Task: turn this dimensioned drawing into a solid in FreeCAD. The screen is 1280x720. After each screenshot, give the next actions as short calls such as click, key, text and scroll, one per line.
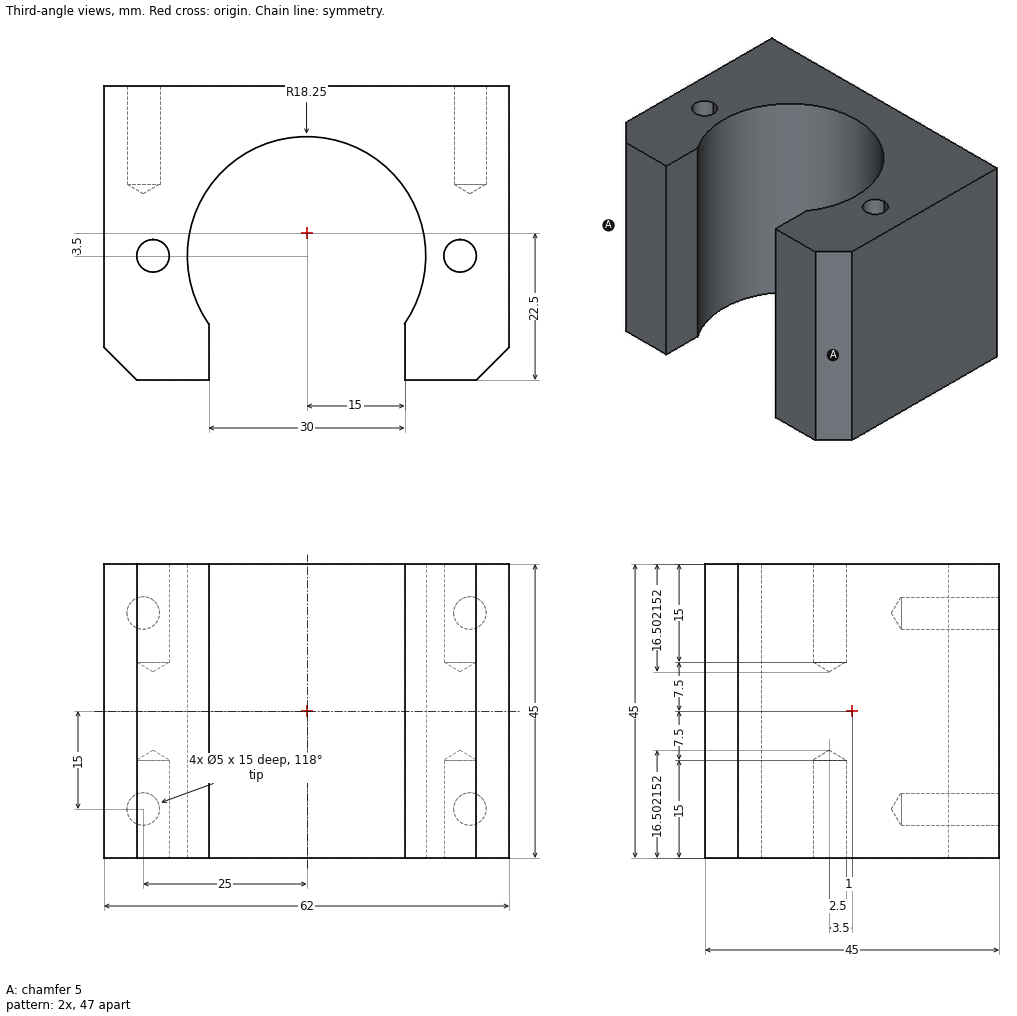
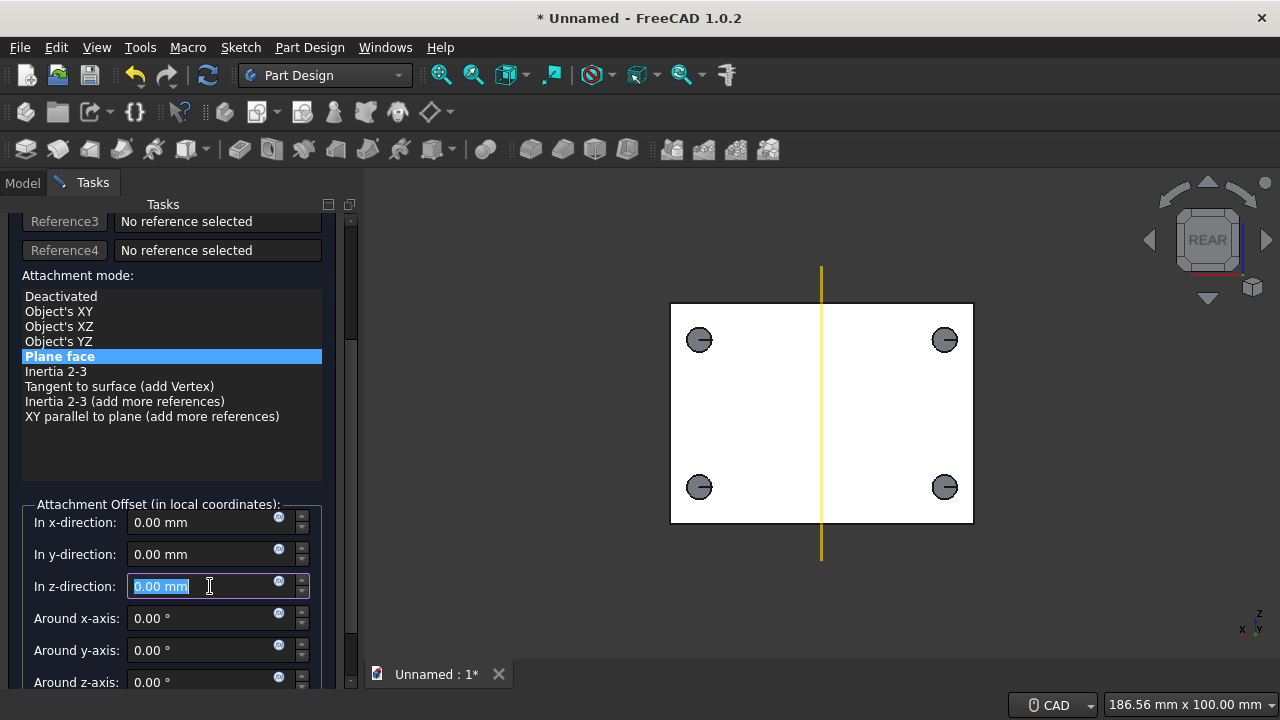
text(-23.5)
key(Tab)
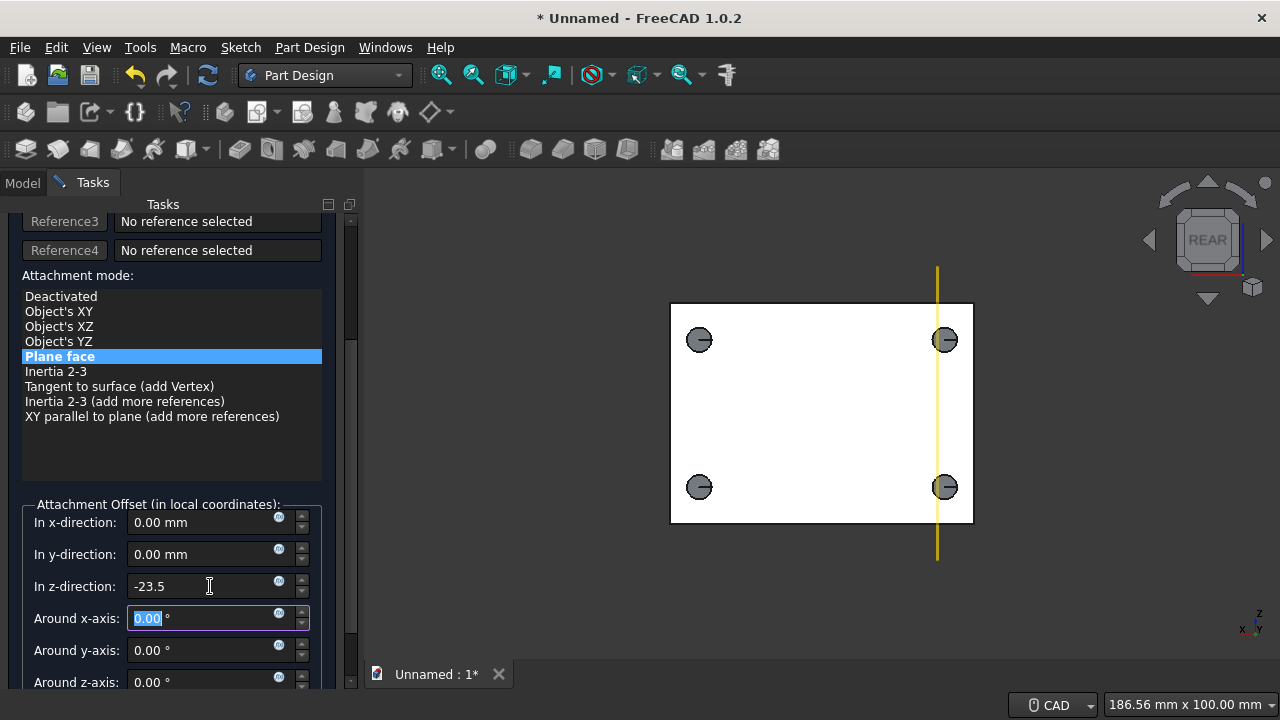
scroll(351, 451, up, 4)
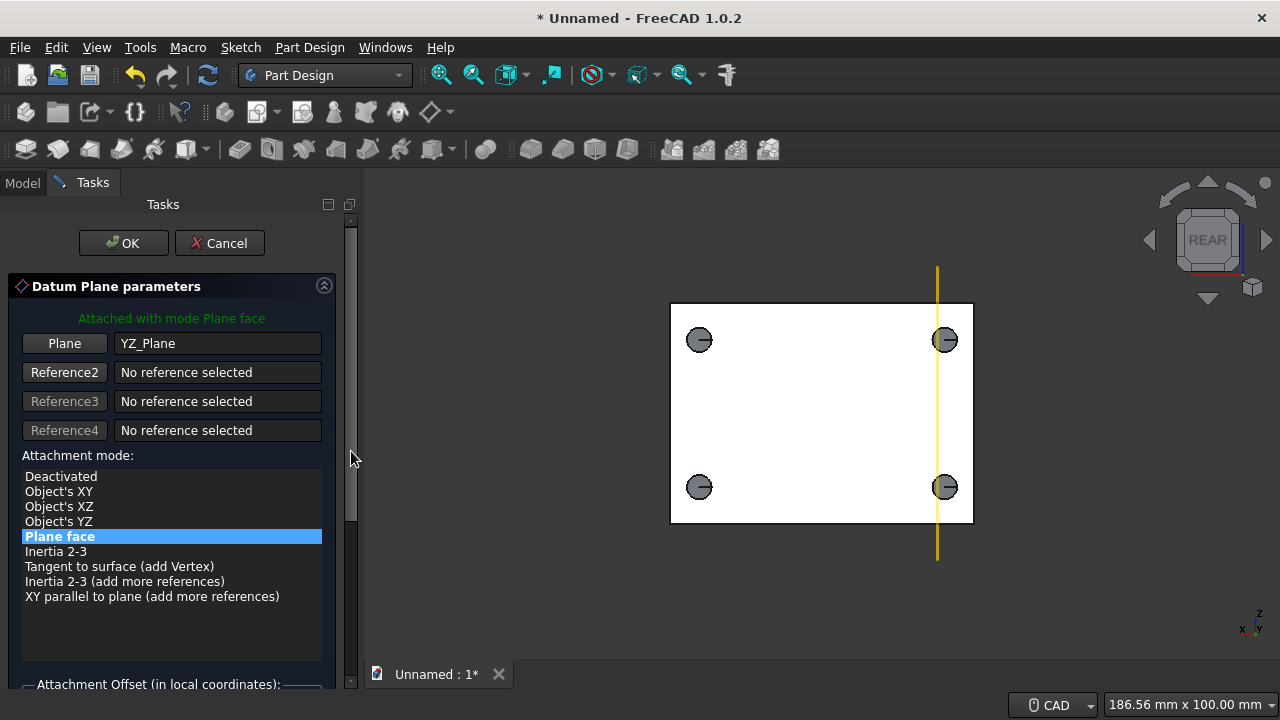
click(124, 243)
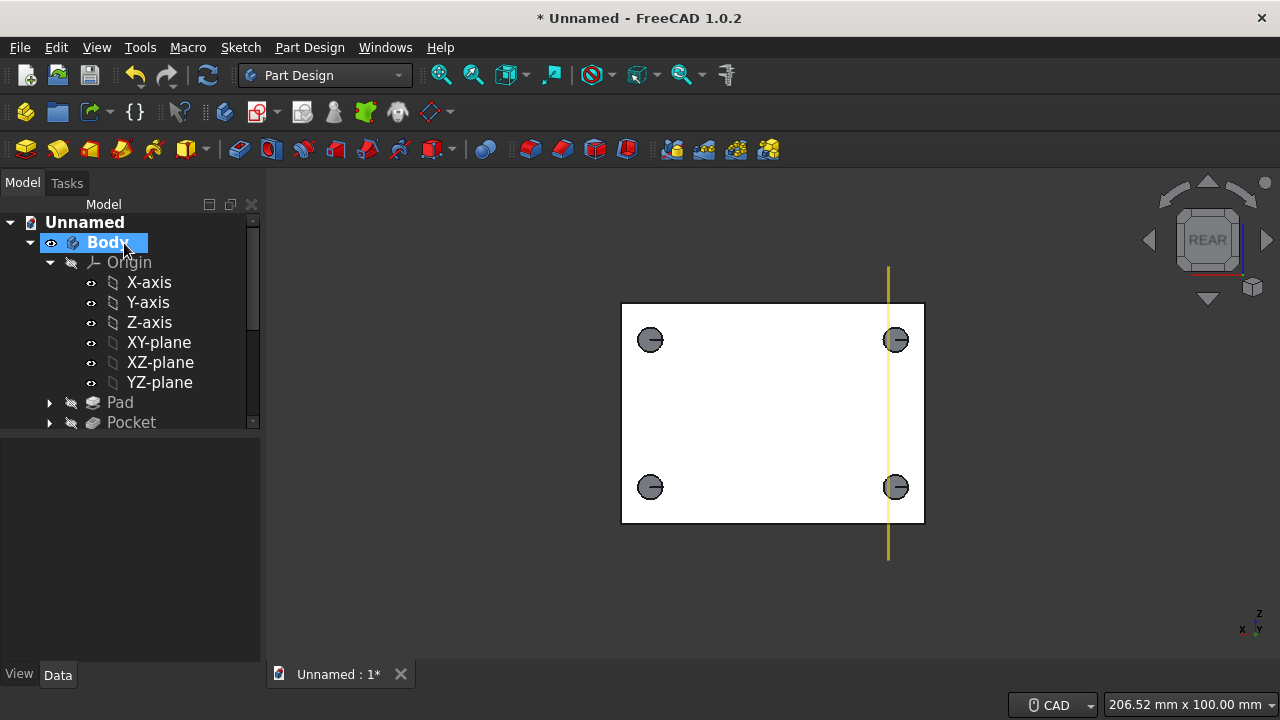
scroll(100, 318, down, 3)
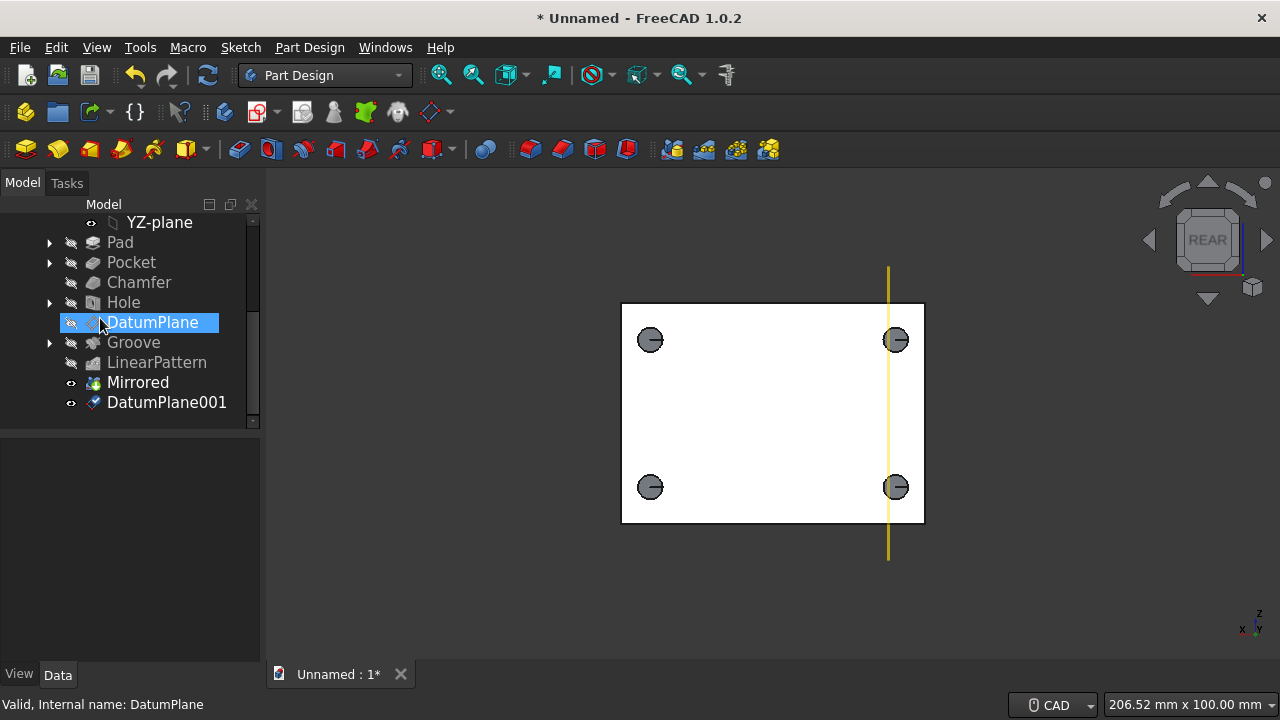
click(116, 403)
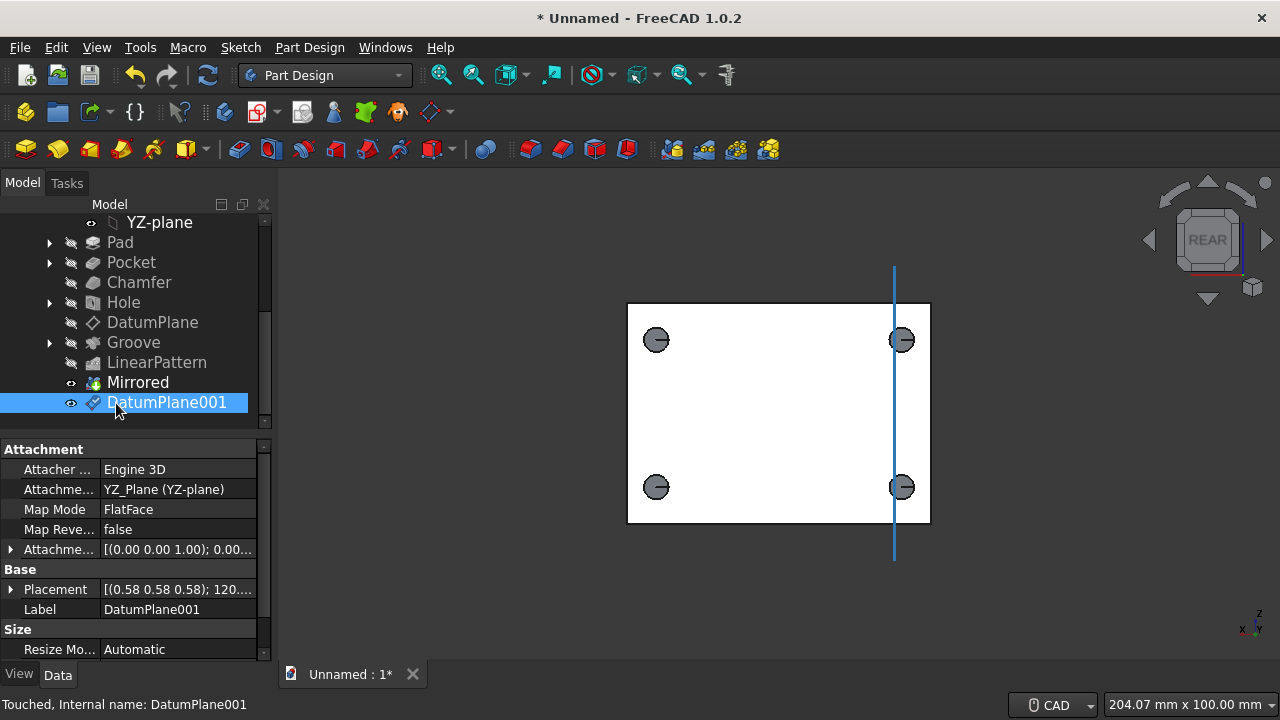
click(258, 112)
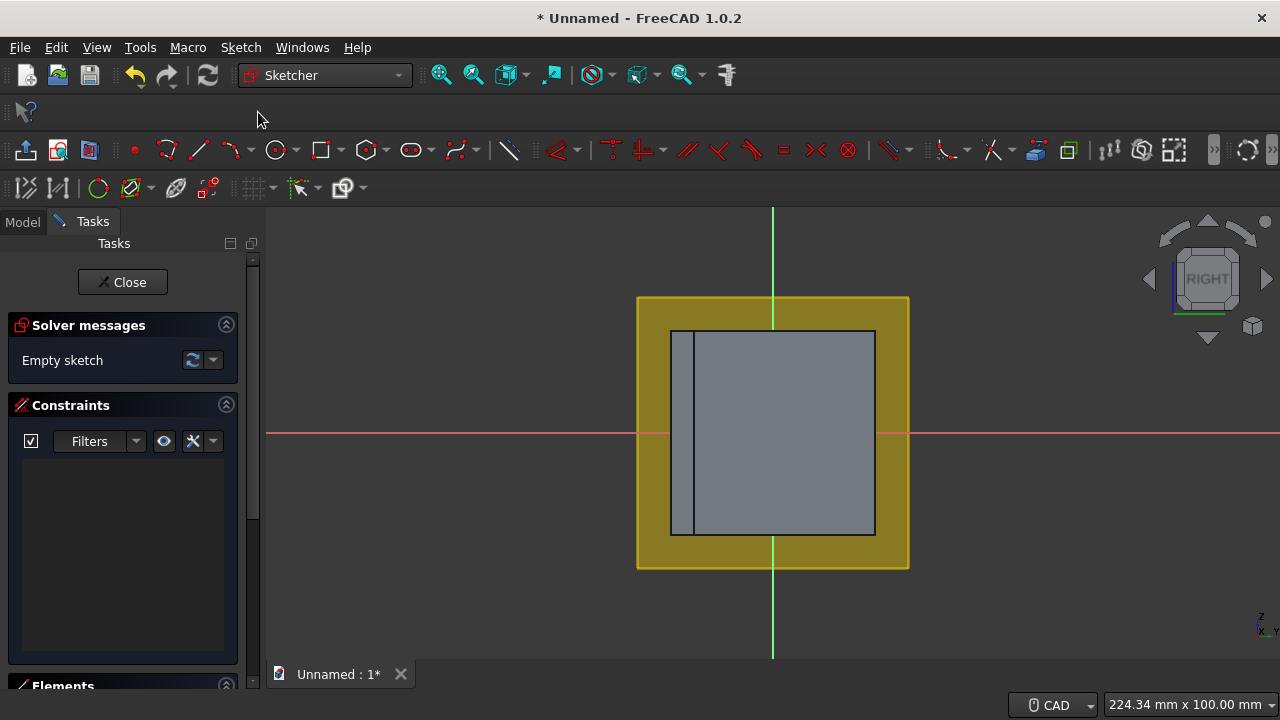
click(90, 150)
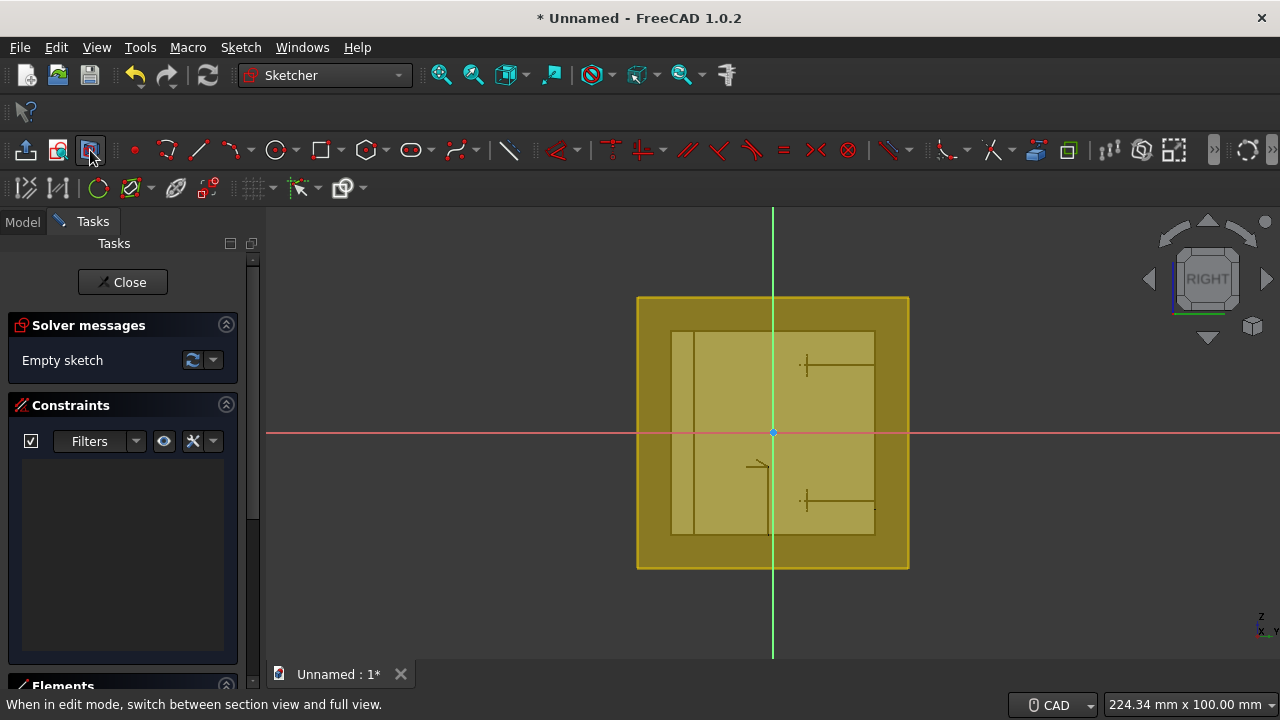
scroll(815, 314, up, 4)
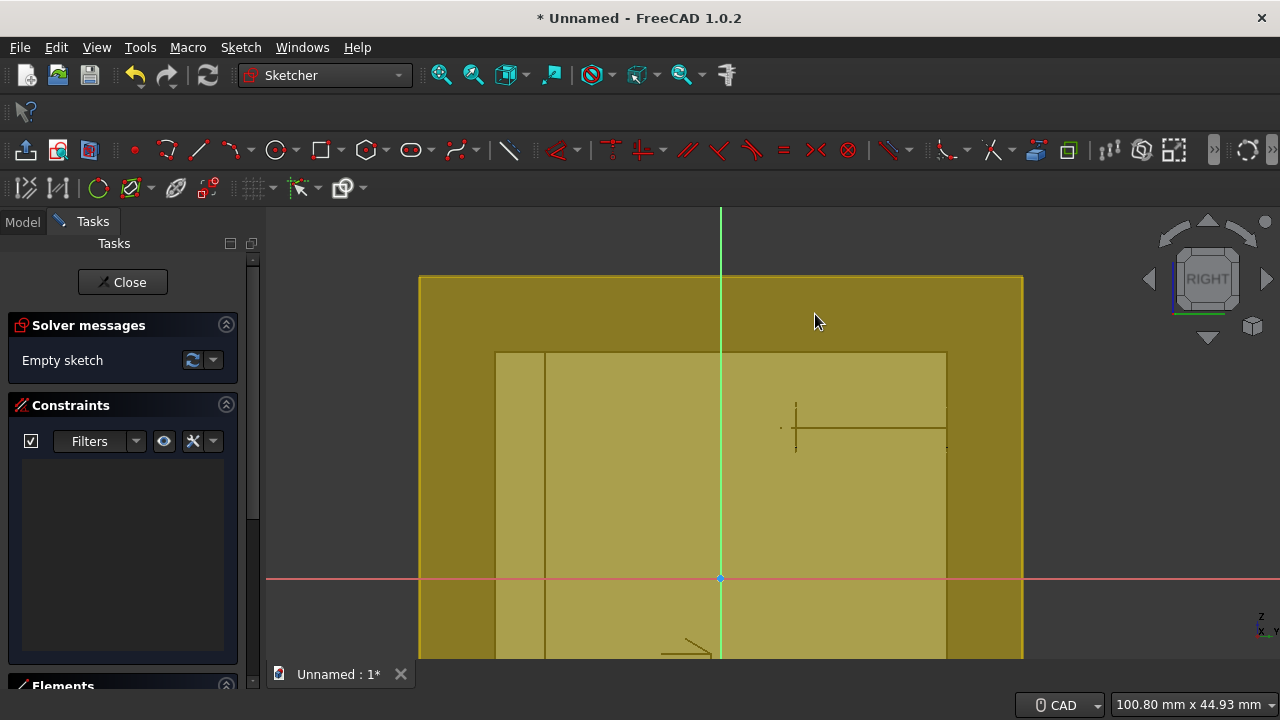
click(168, 150)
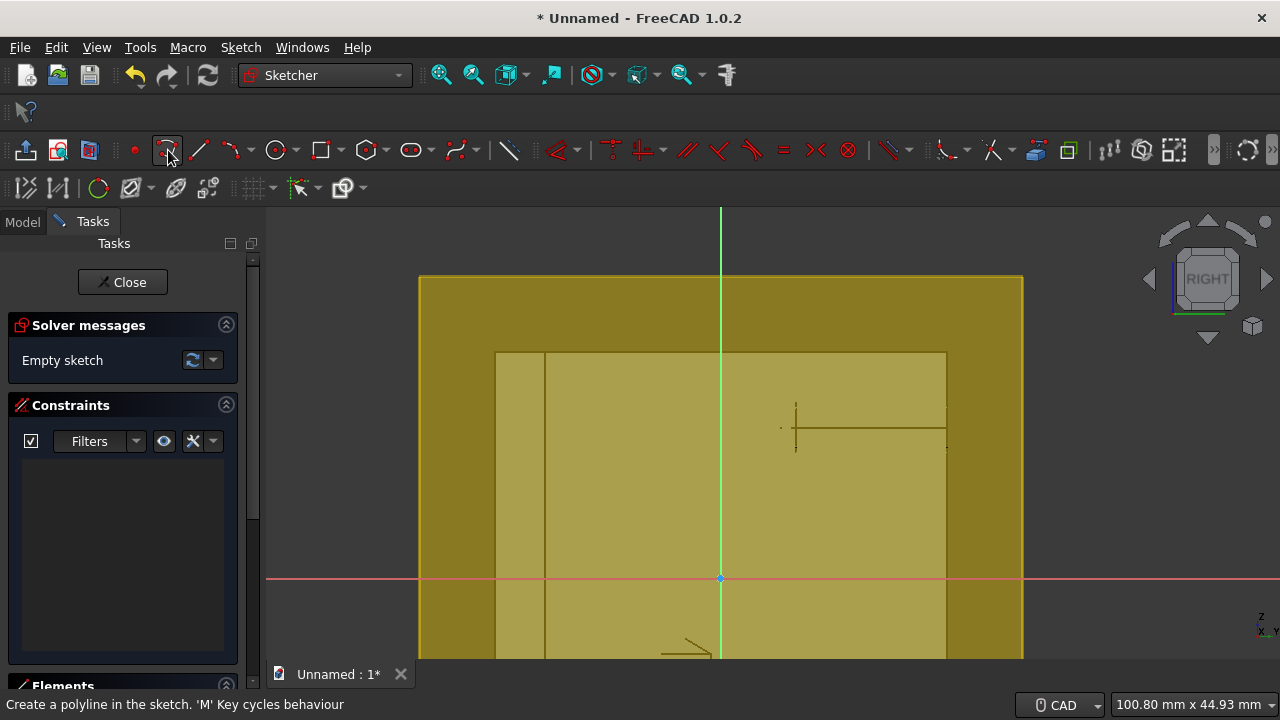
click(686, 518)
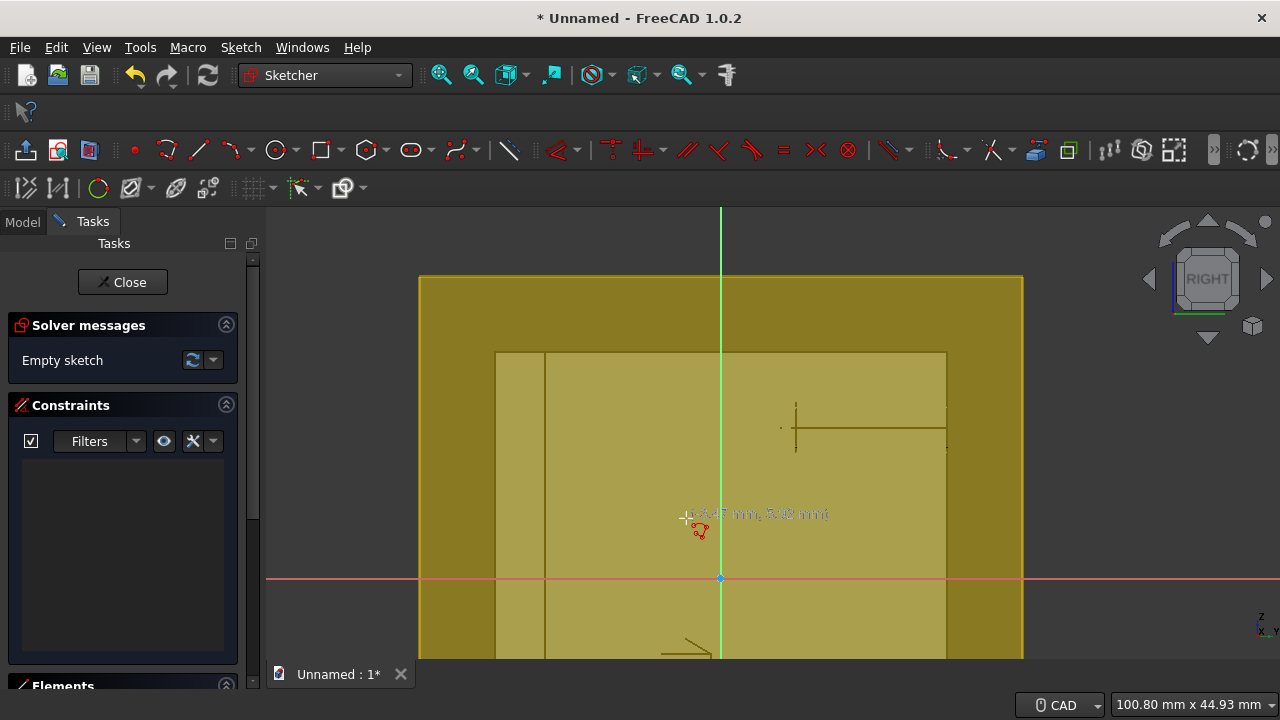
scroll(711, 503, up, 3)